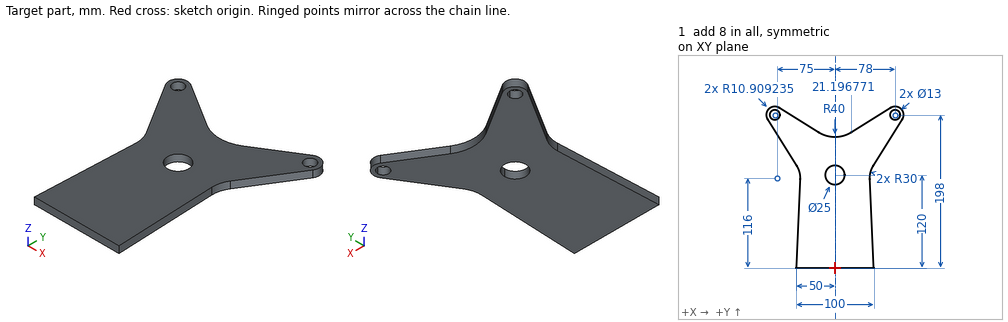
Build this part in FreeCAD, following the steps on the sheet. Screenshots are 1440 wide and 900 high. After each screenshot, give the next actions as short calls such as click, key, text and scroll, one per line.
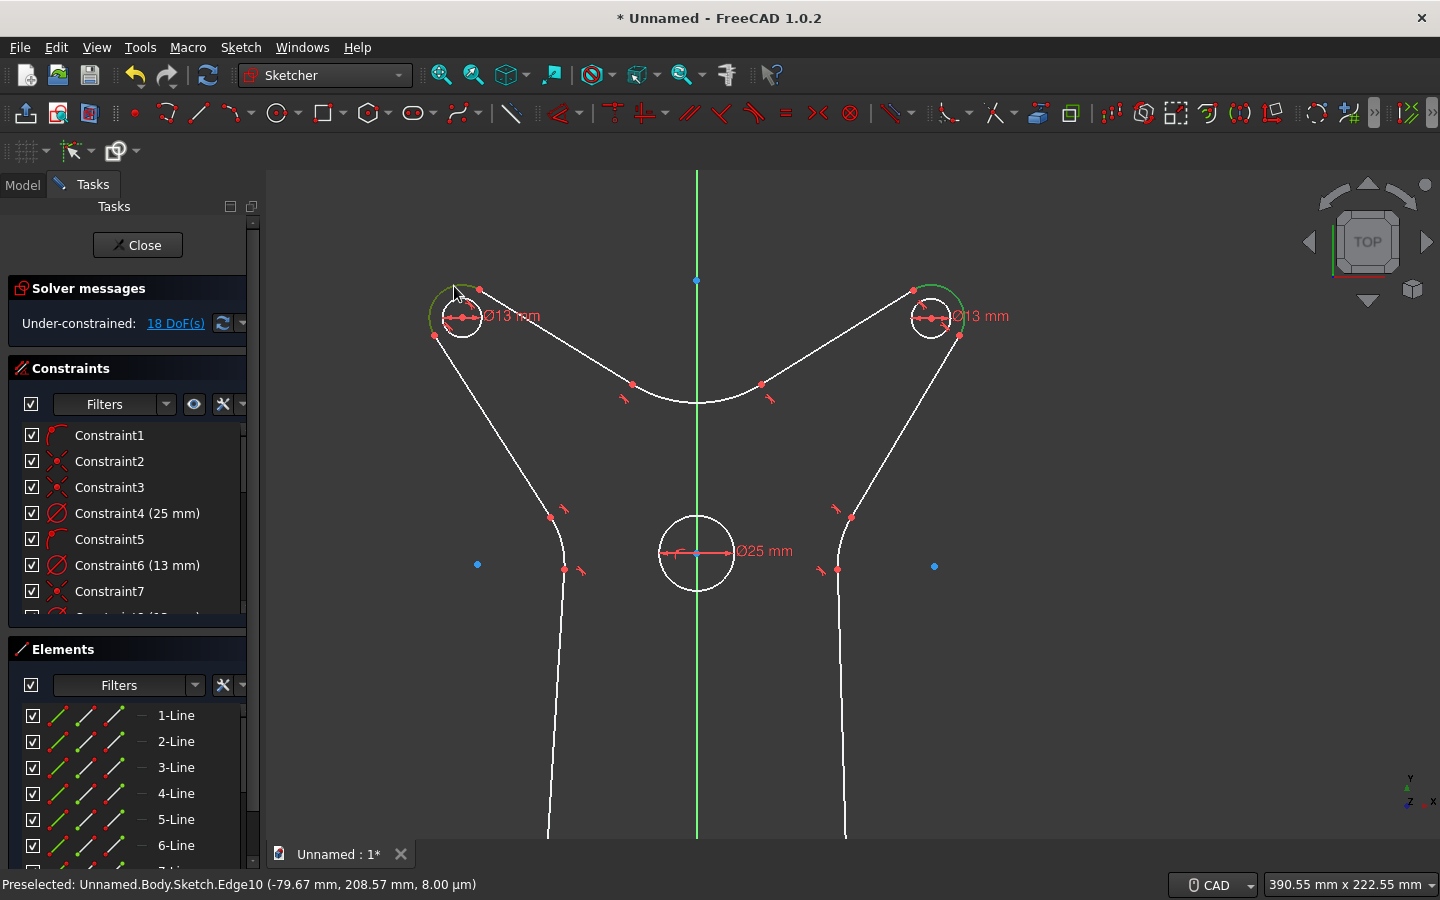
click(786, 114)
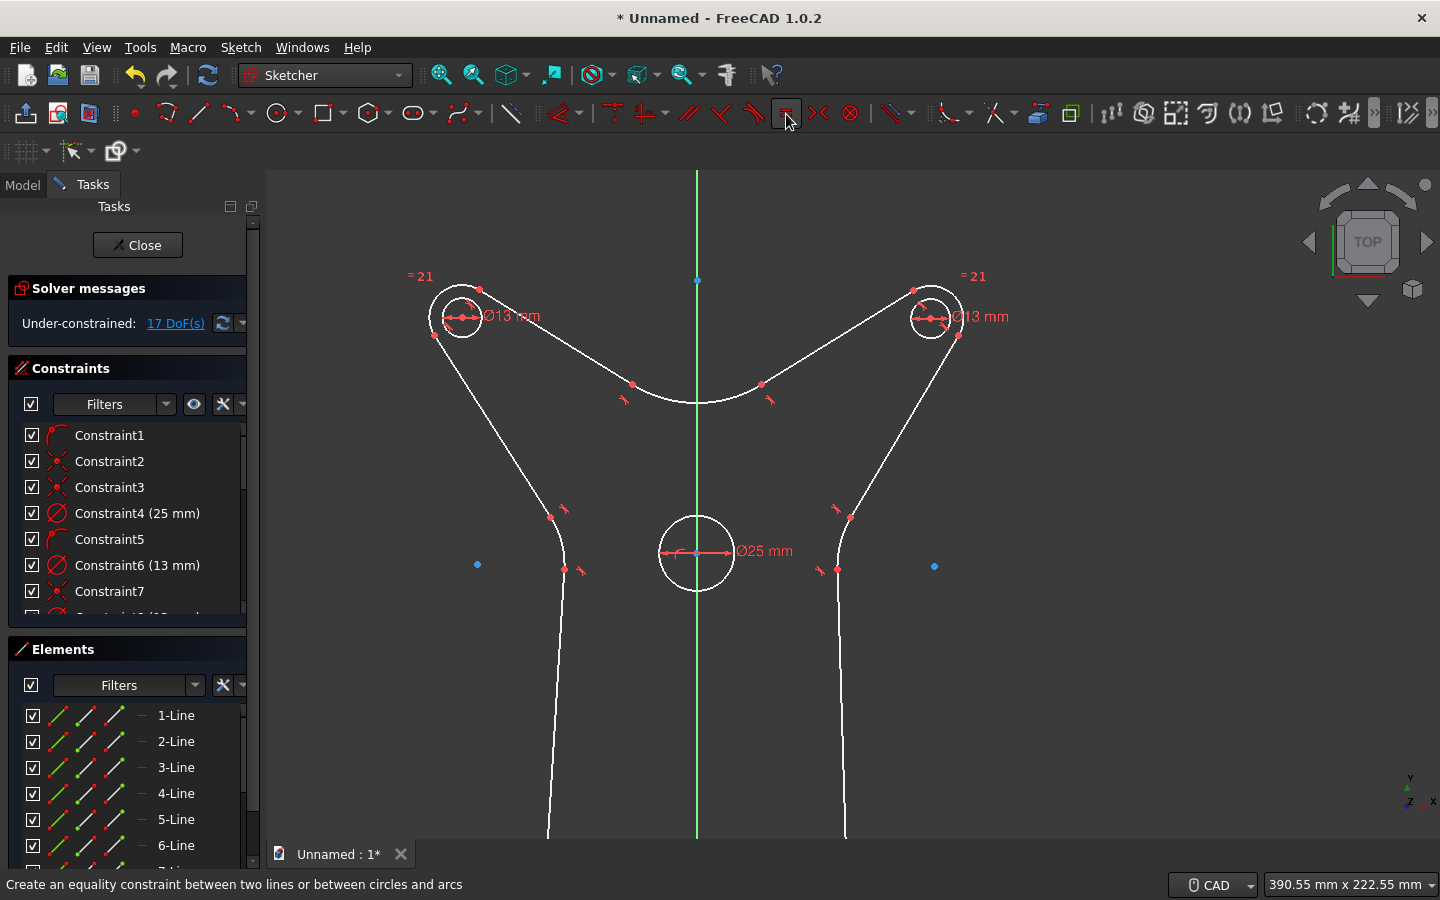
click(564, 553)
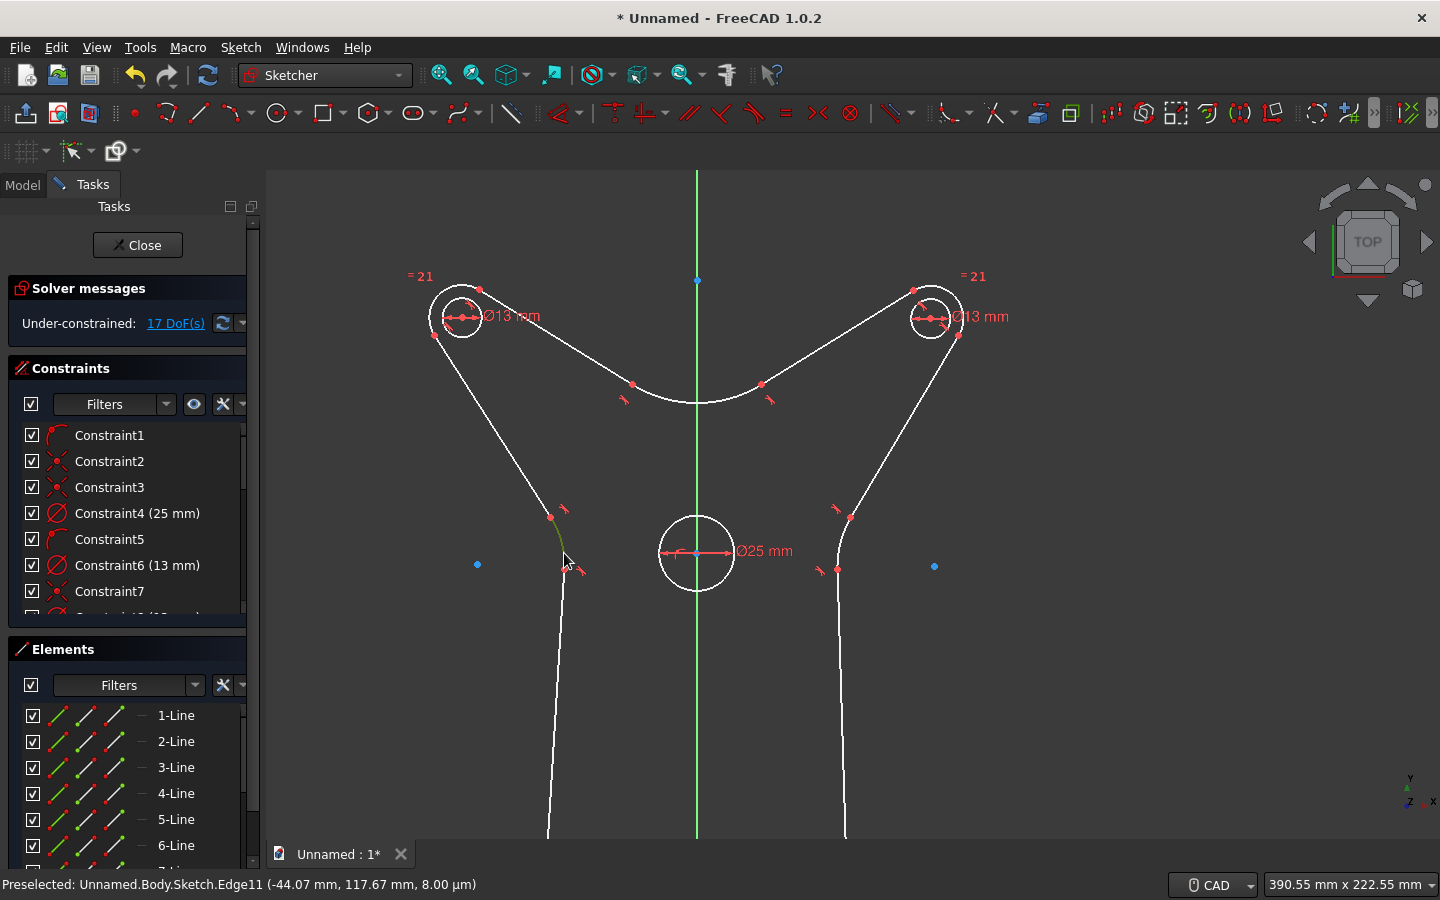
click(844, 532)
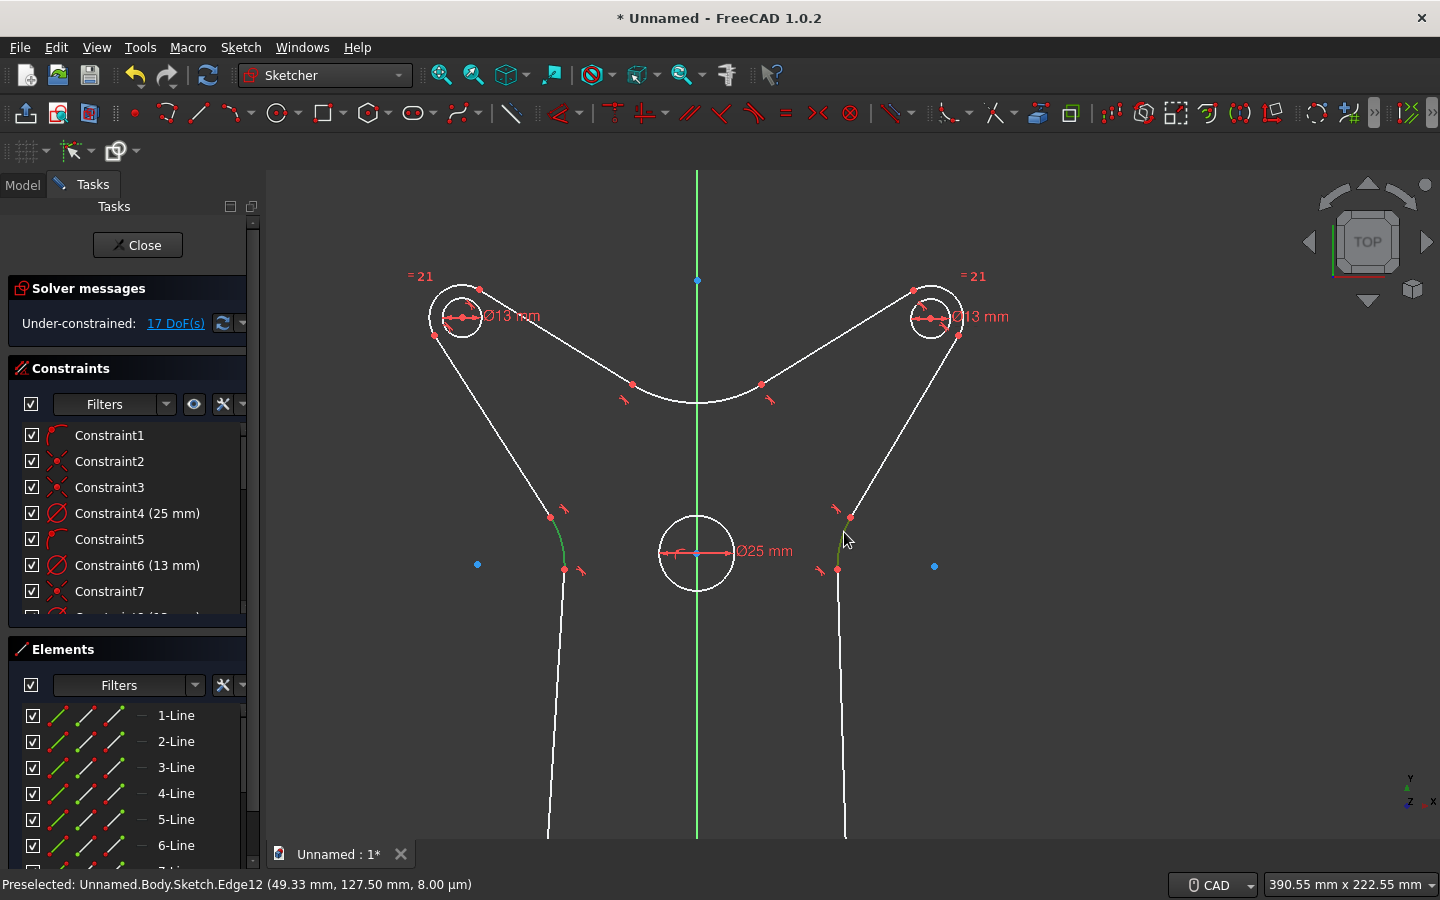
click(786, 114)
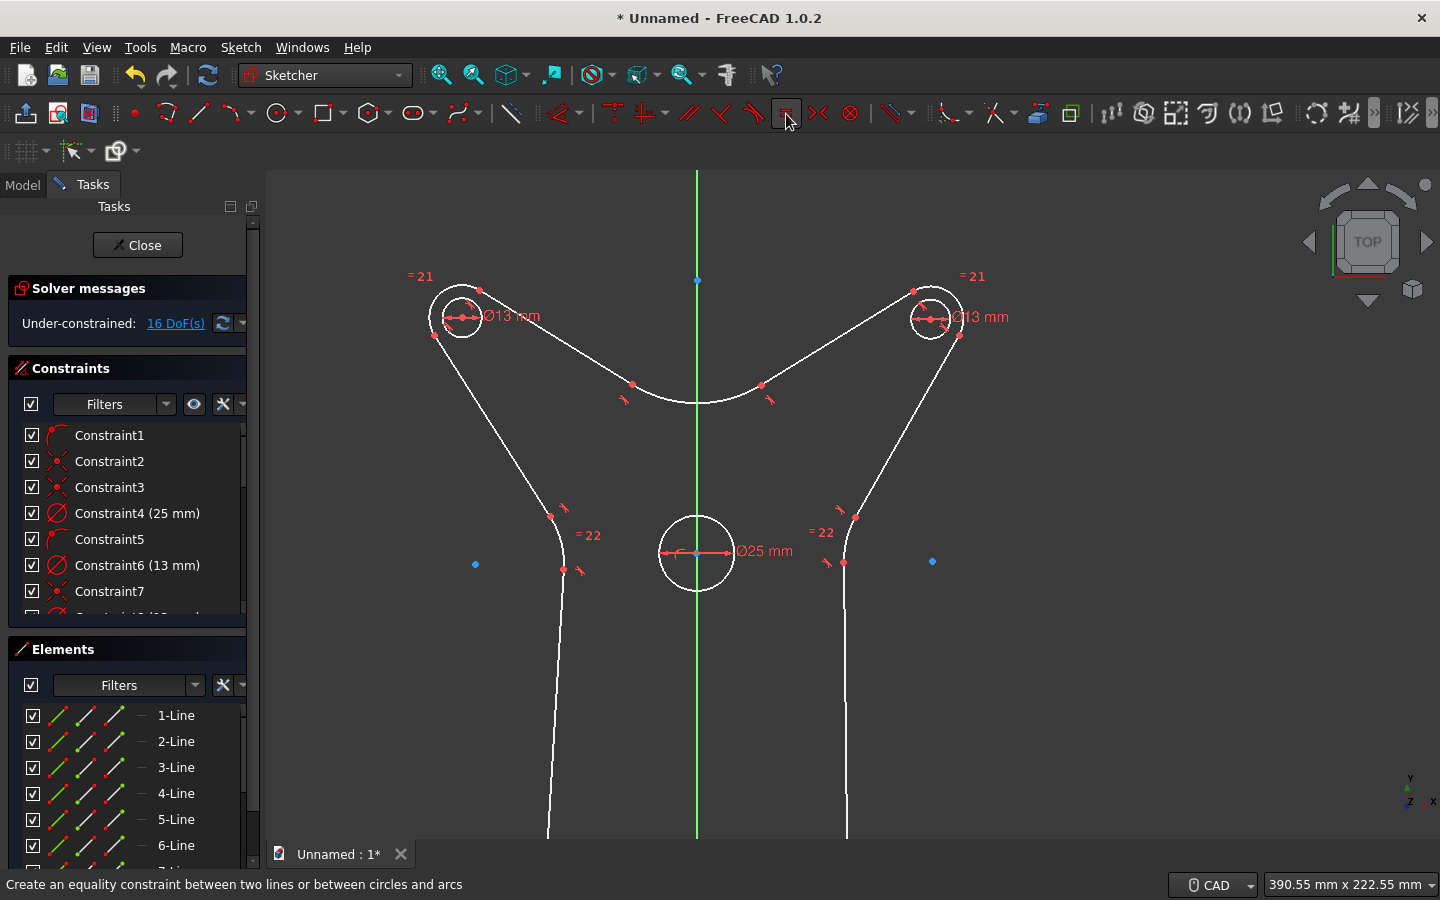
click(697, 281)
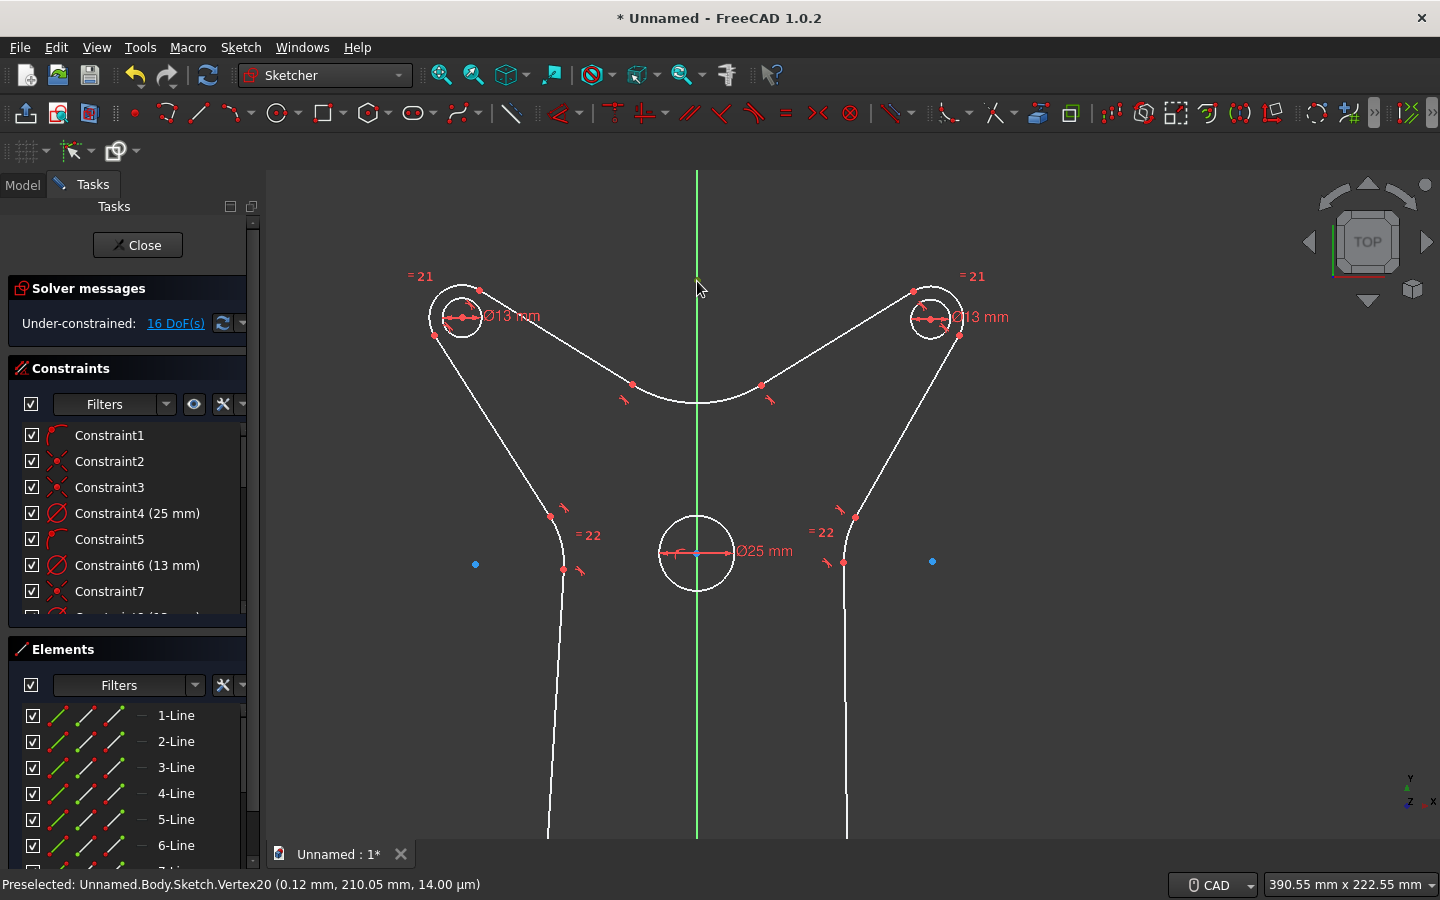
click(697, 767)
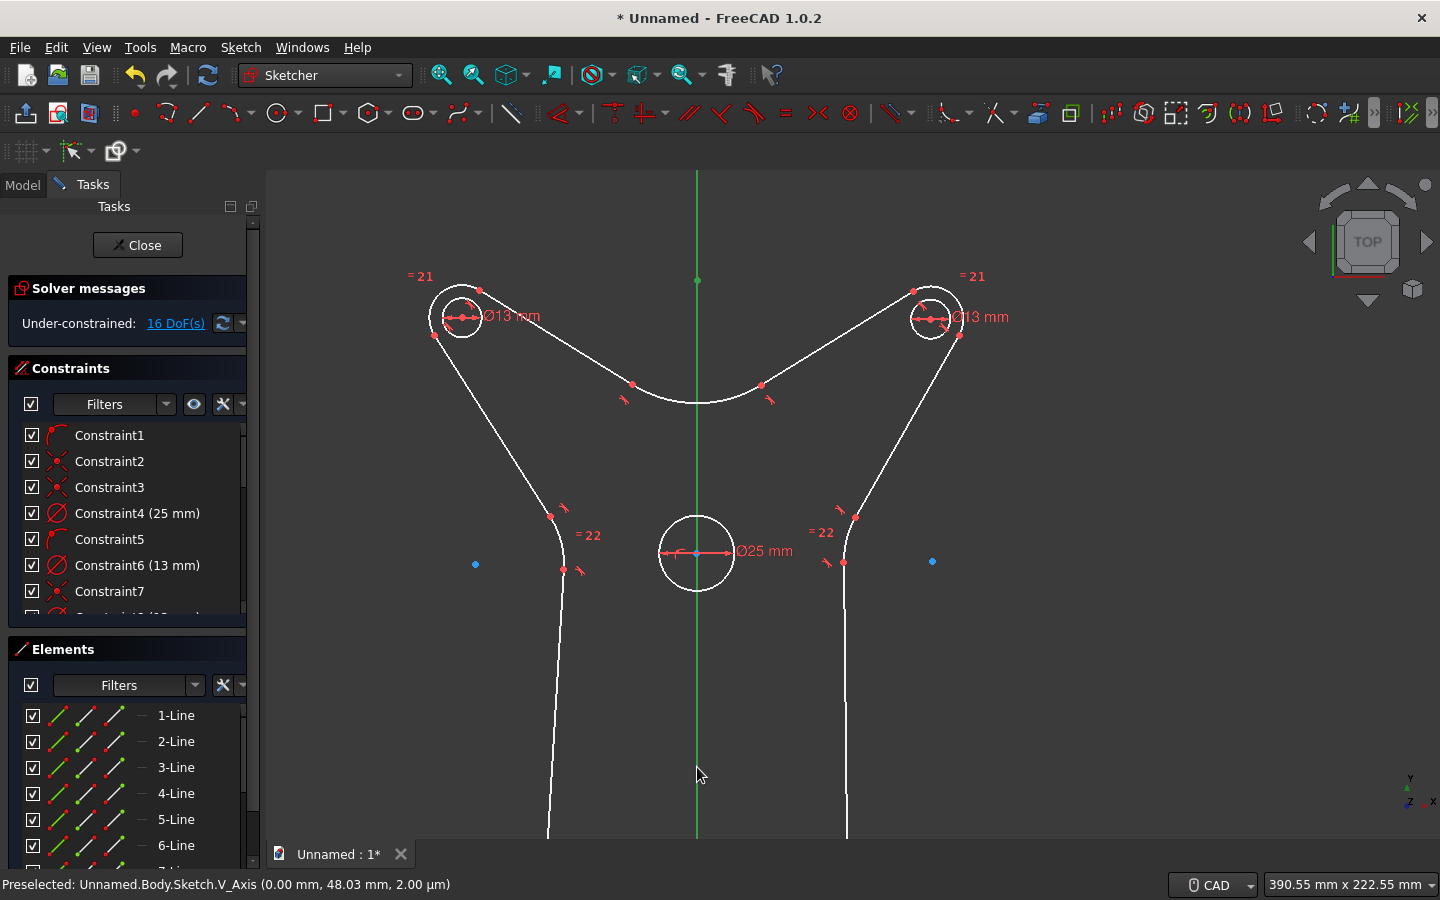
click(614, 114)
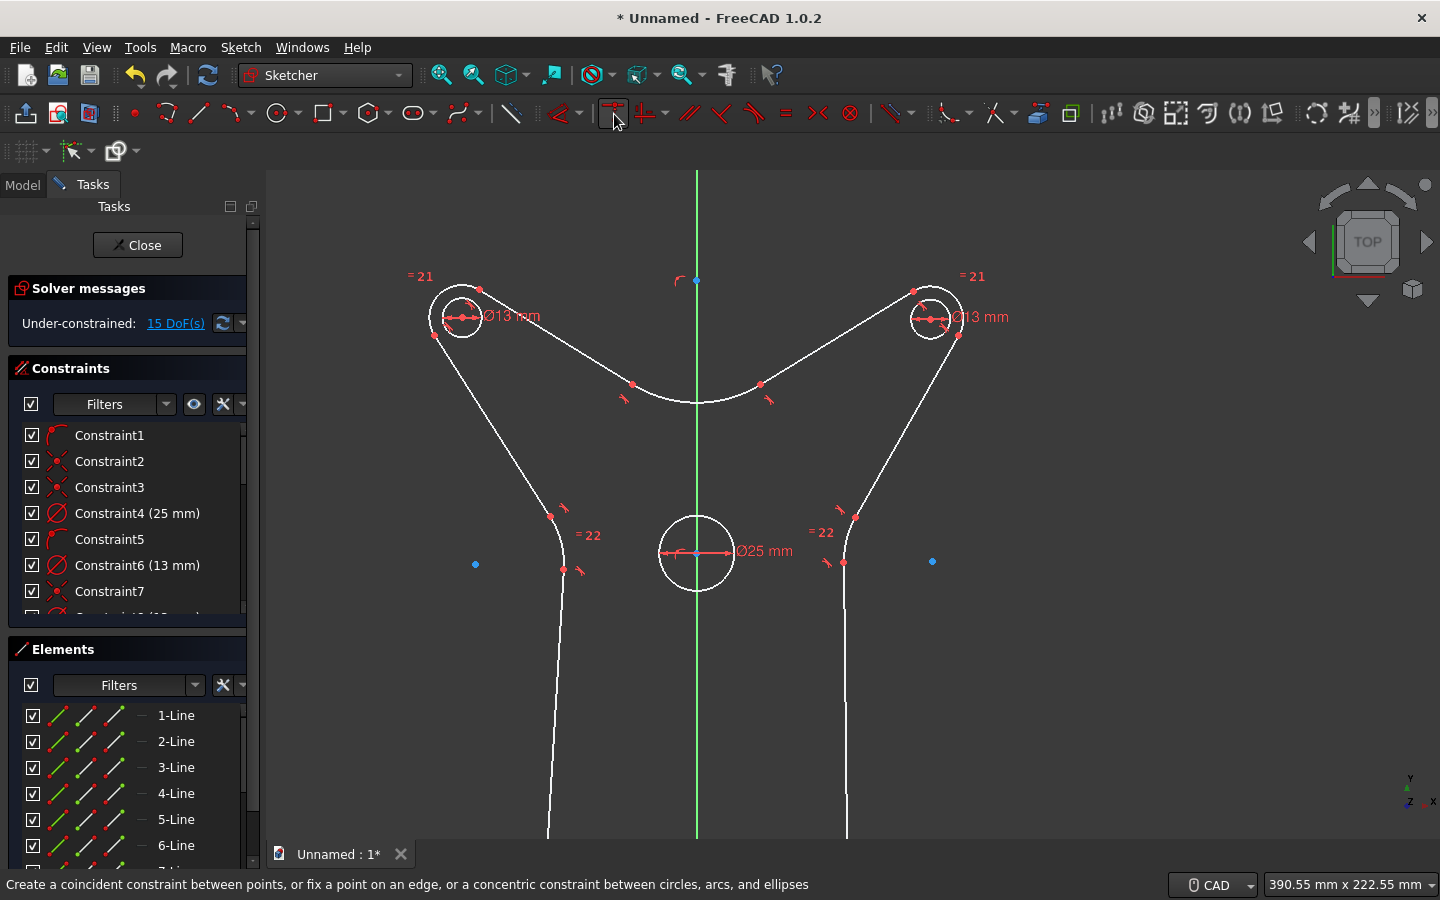
click(931, 319)